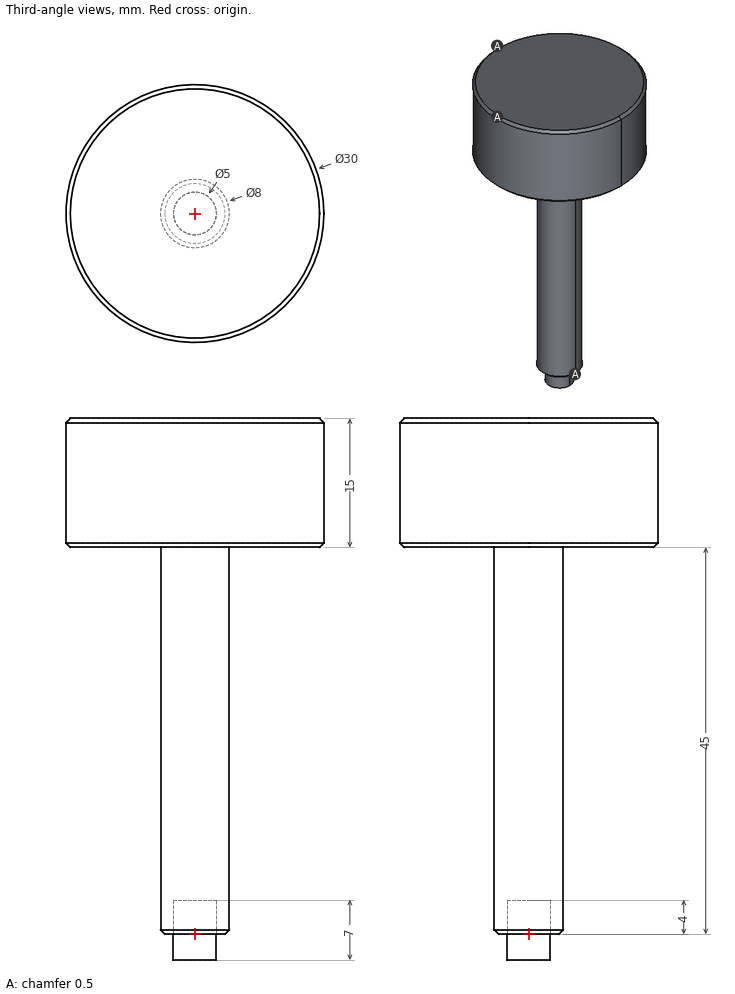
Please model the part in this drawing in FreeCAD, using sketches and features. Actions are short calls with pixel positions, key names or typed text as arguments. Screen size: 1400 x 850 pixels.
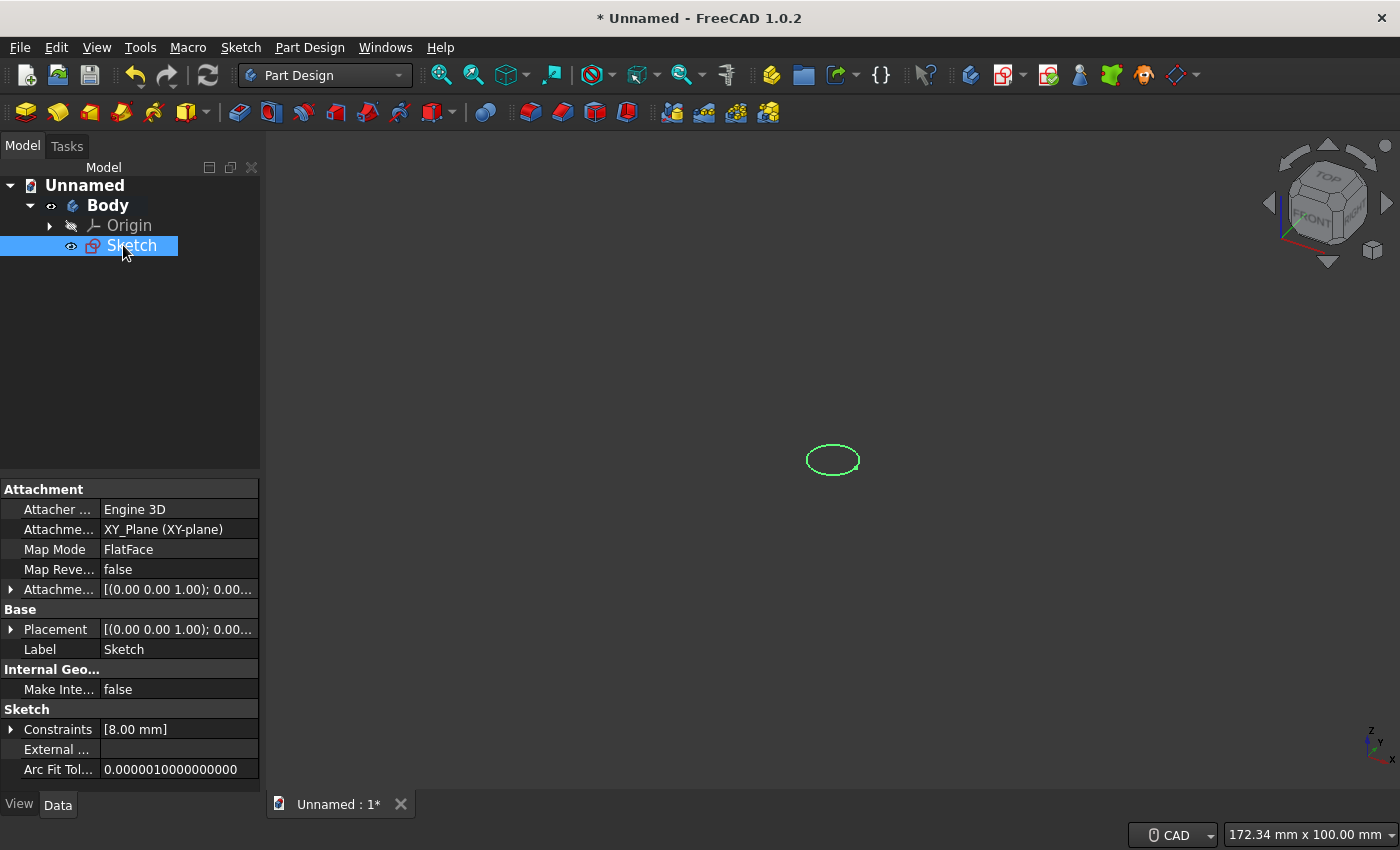
click(26, 112)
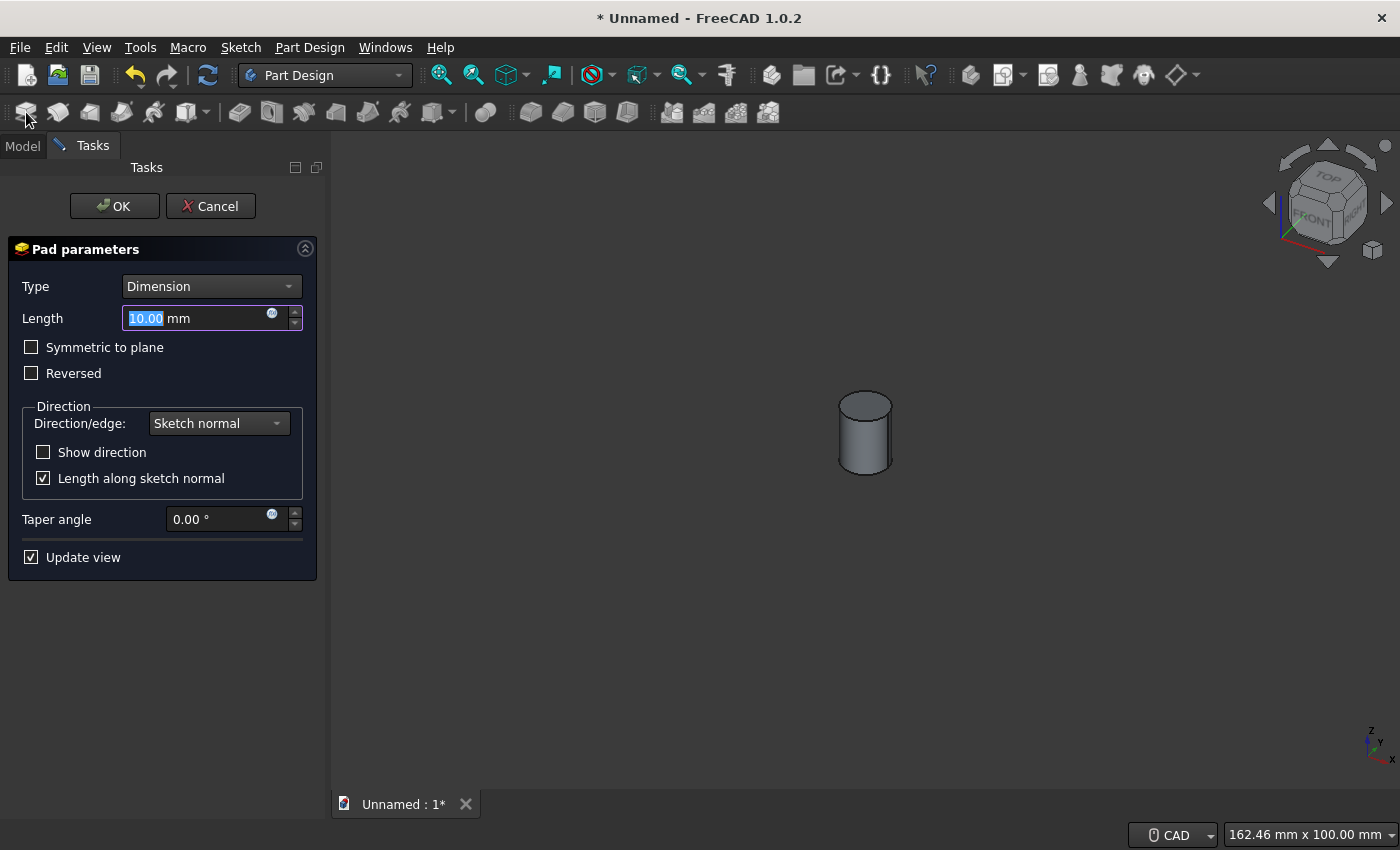
text(45)
key(Tab)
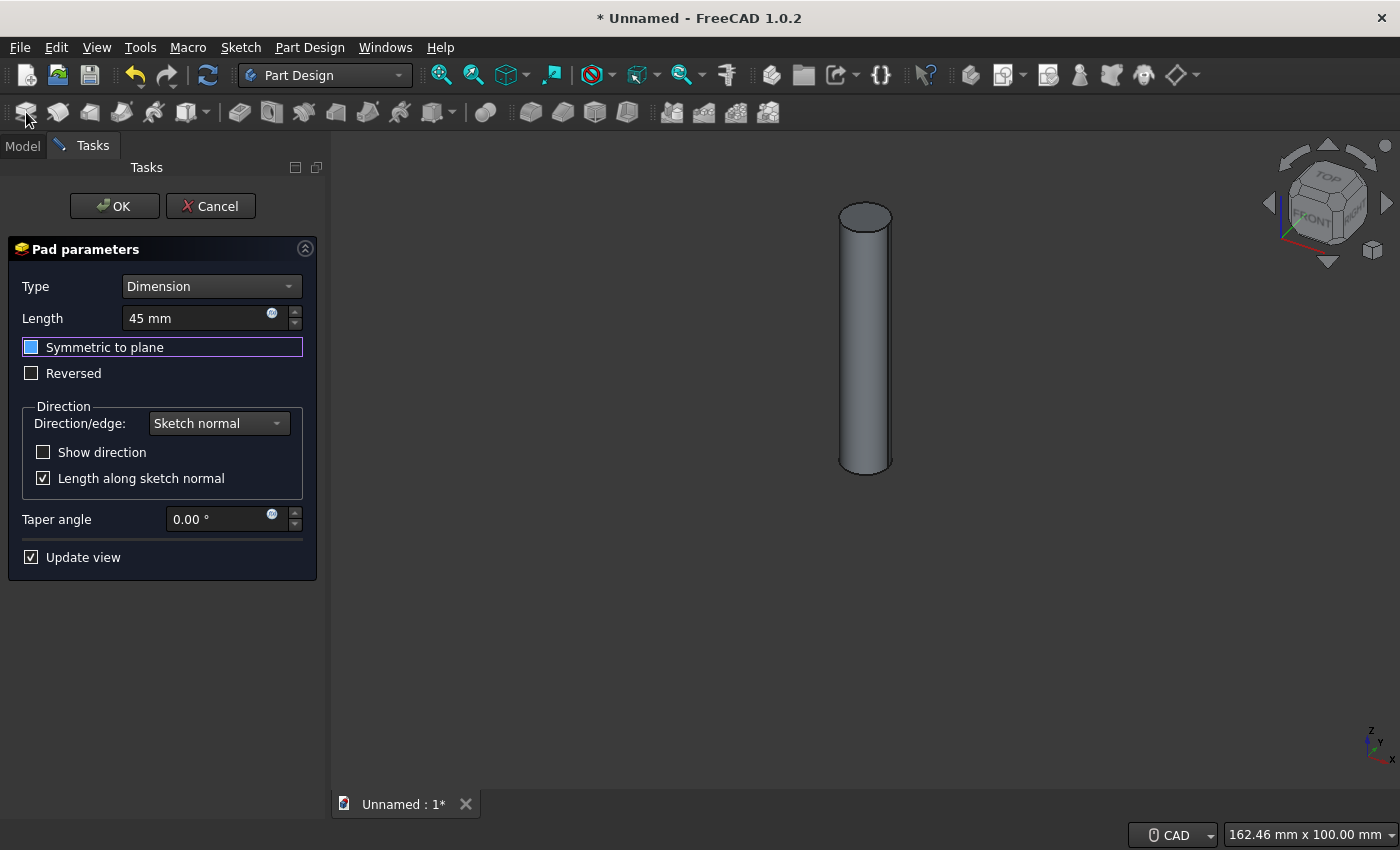
click(115, 206)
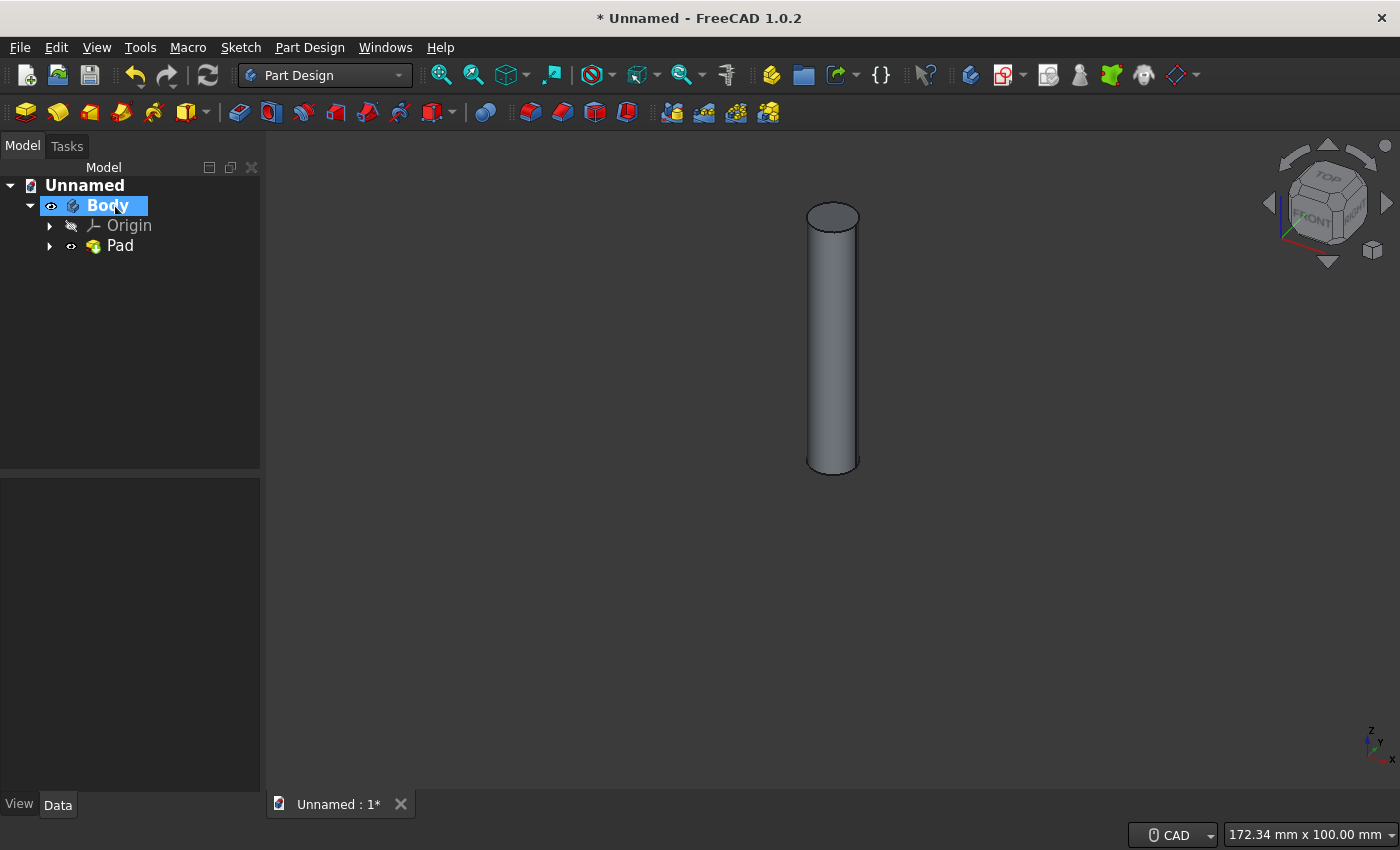
click(442, 76)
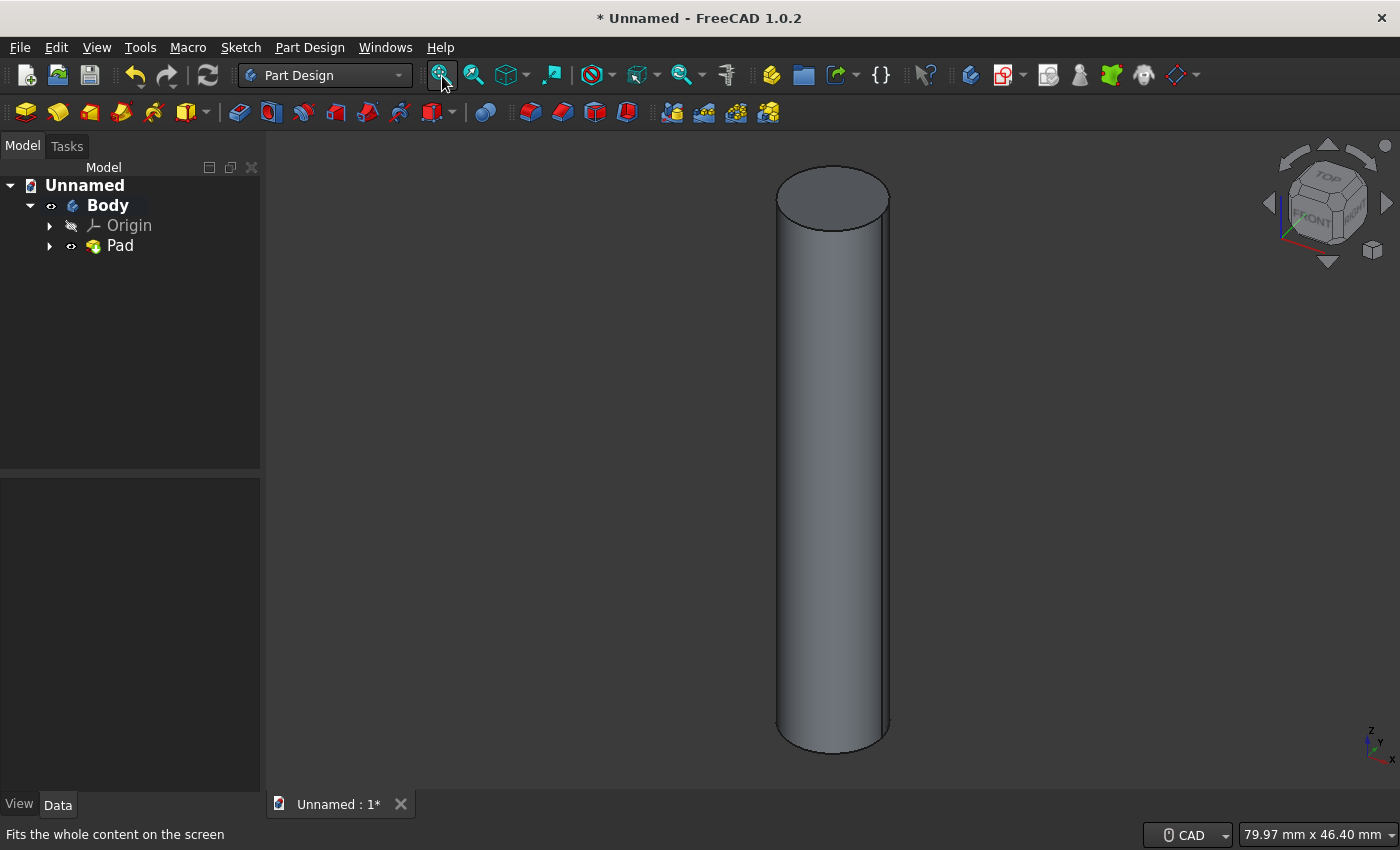
click(833, 198)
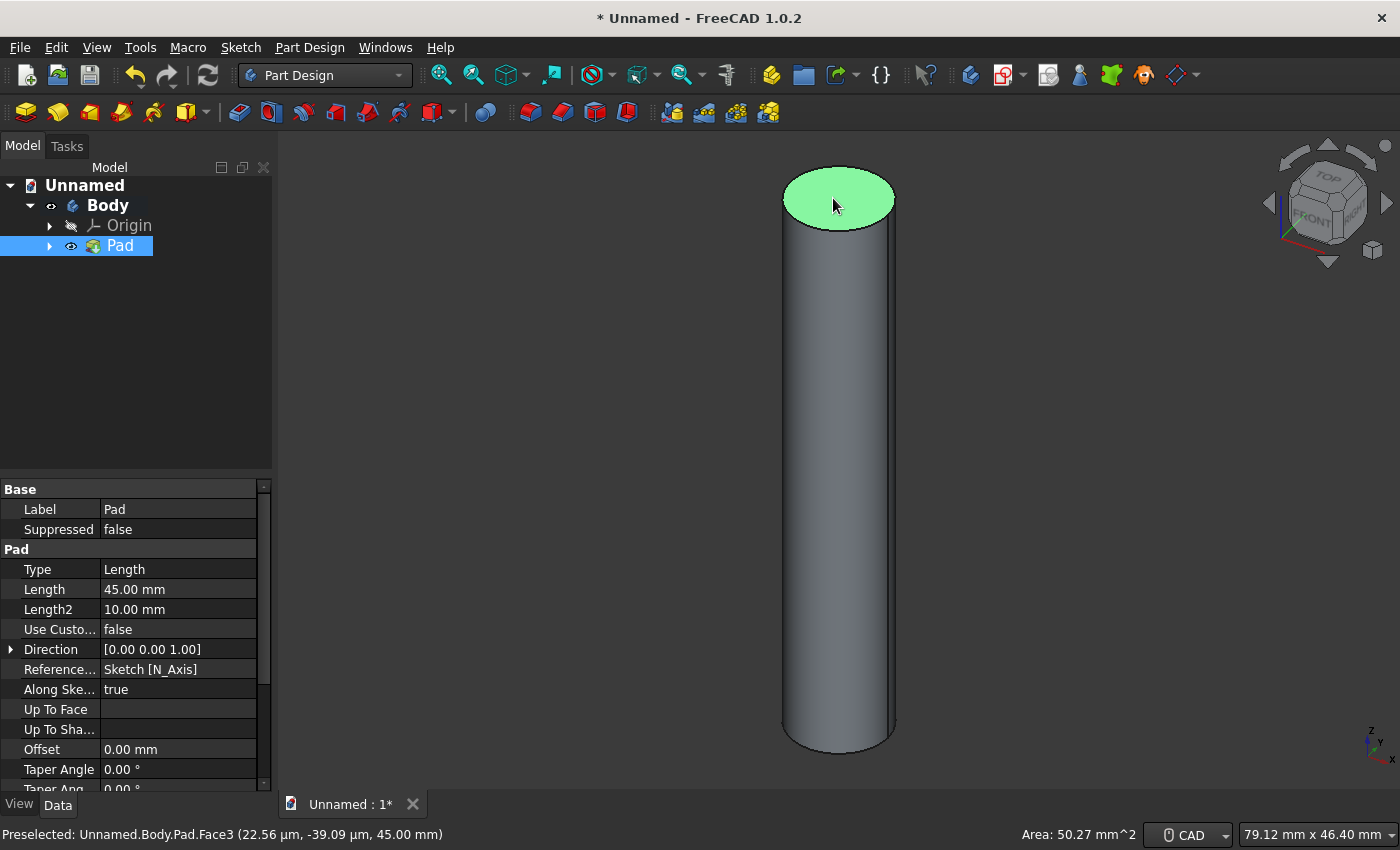
click(1004, 76)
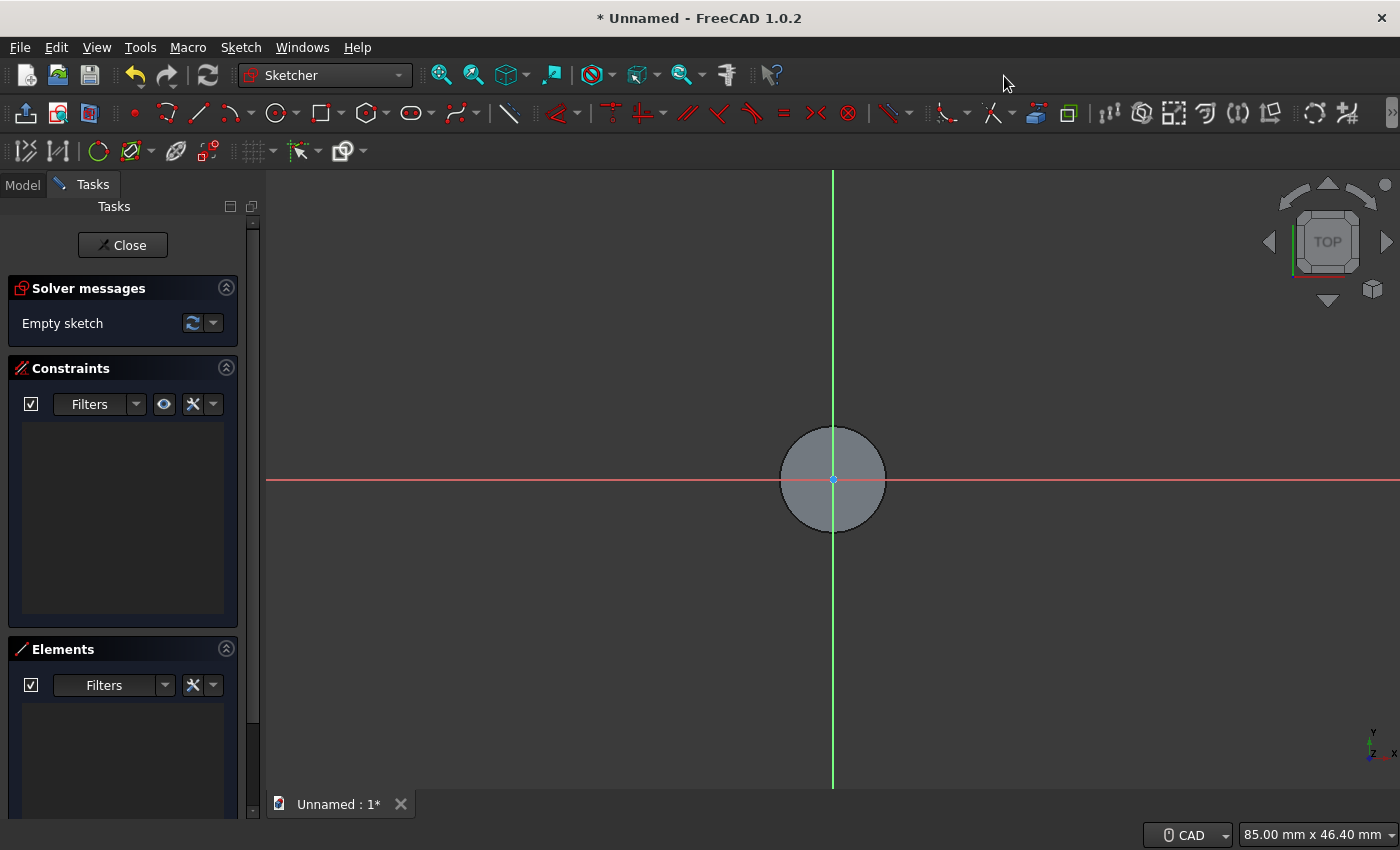
click(276, 114)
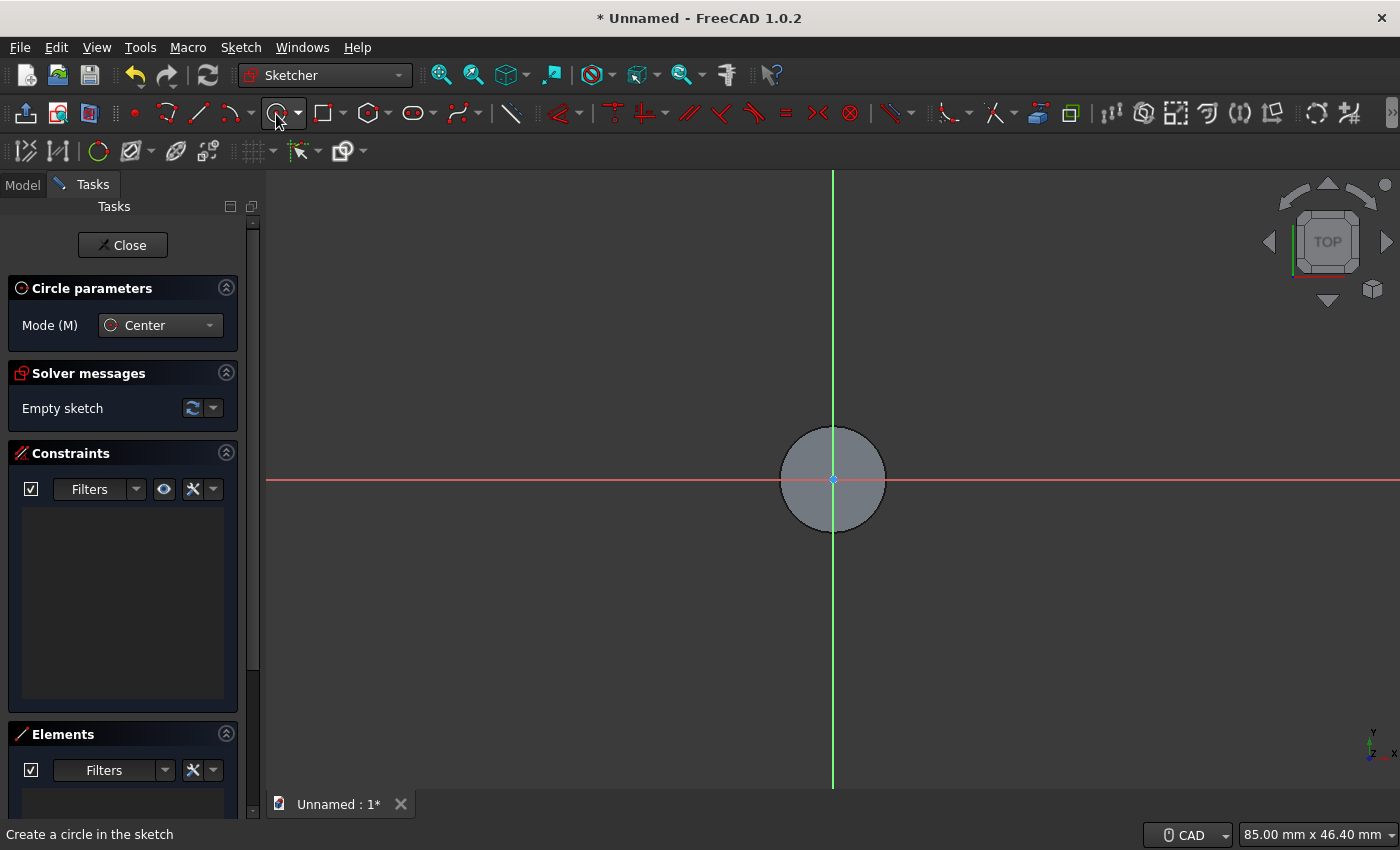
click(833, 480)
move(974, 338)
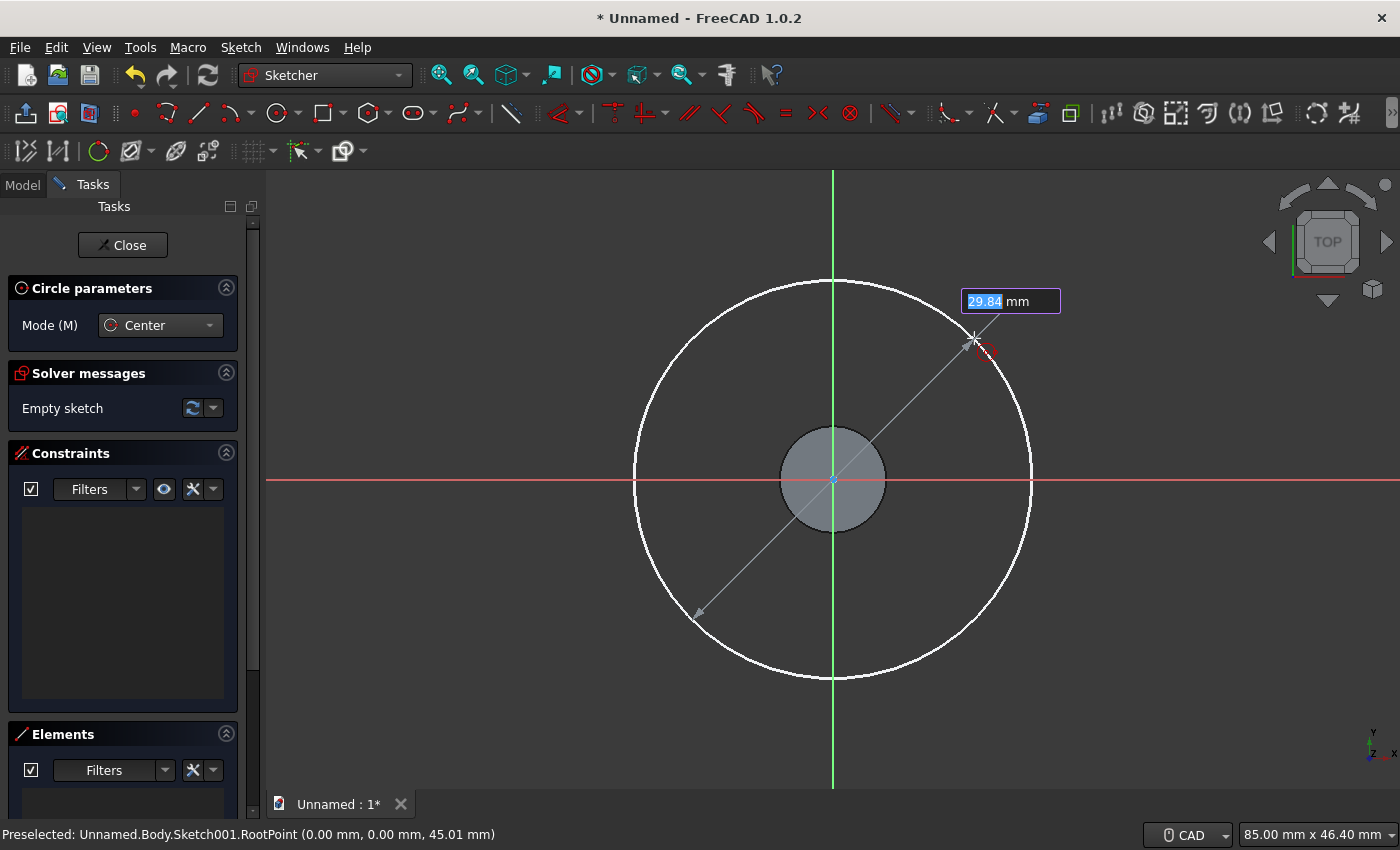
text(30)
key(Return)
key(Escape)